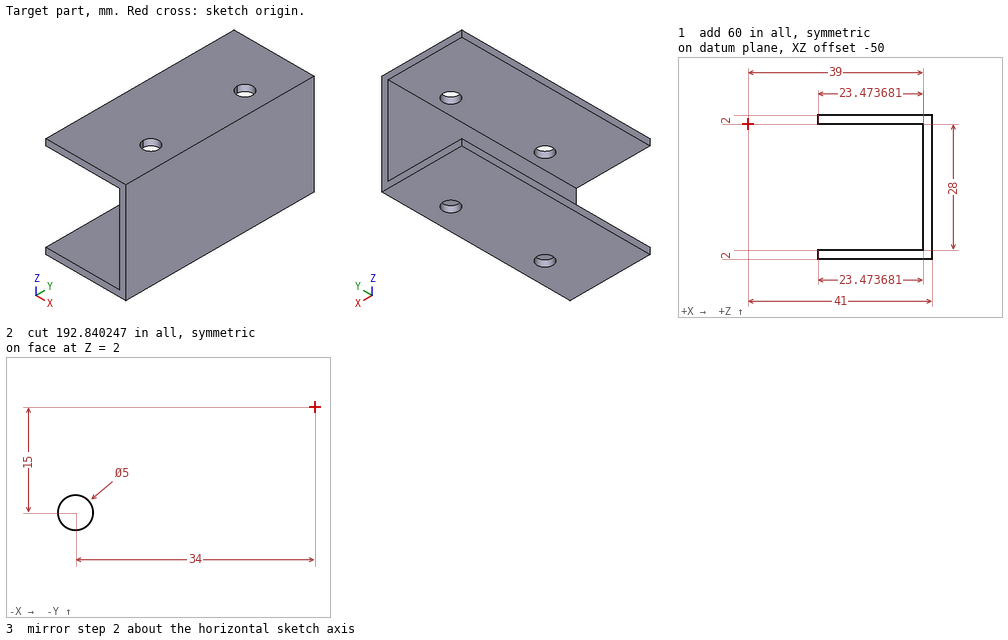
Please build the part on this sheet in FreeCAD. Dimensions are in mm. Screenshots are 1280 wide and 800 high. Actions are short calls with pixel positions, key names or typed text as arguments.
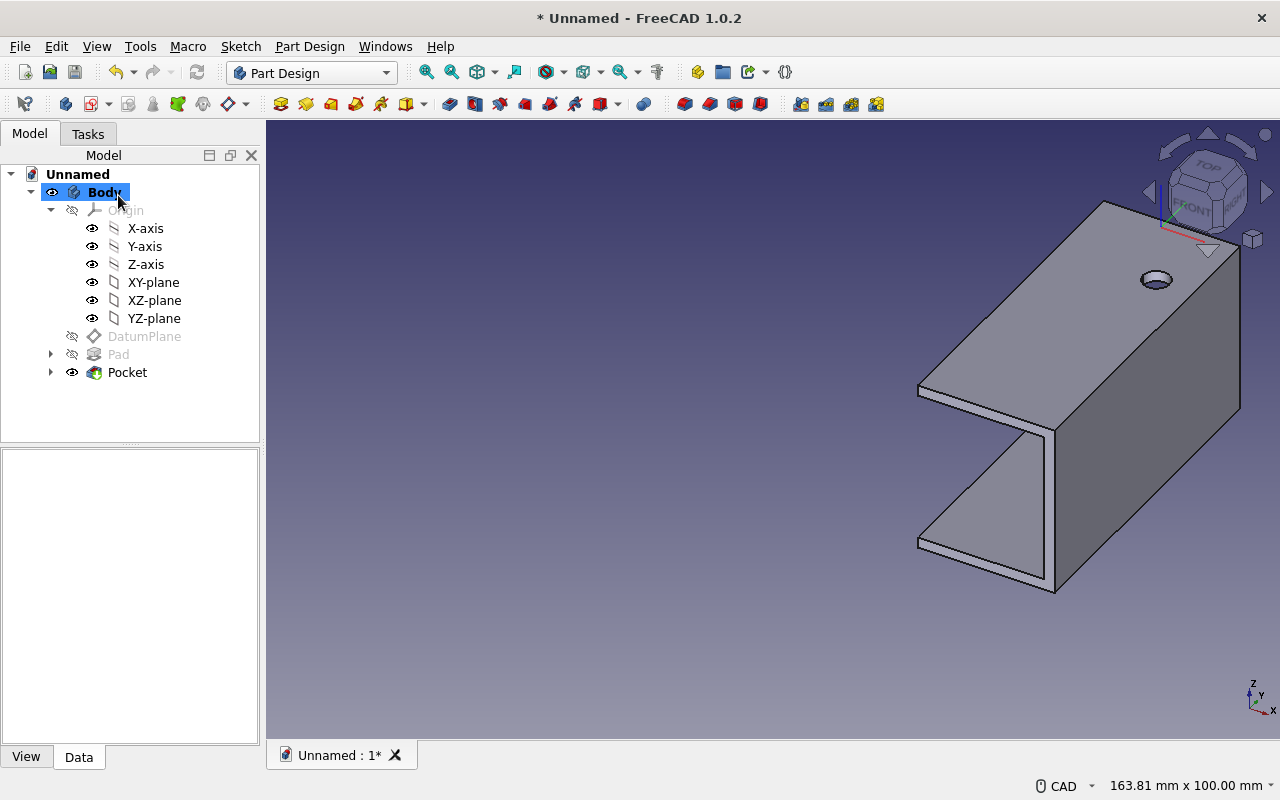
click(117, 372)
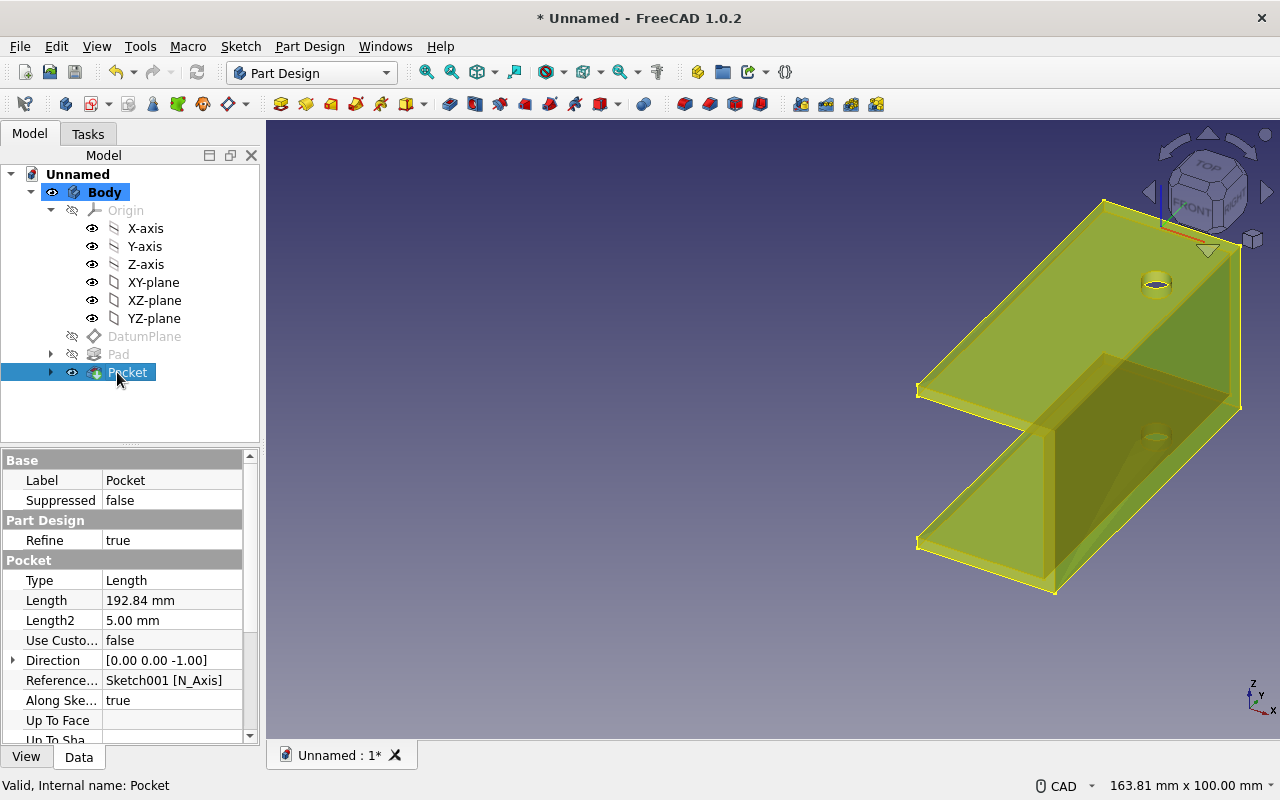
click(801, 104)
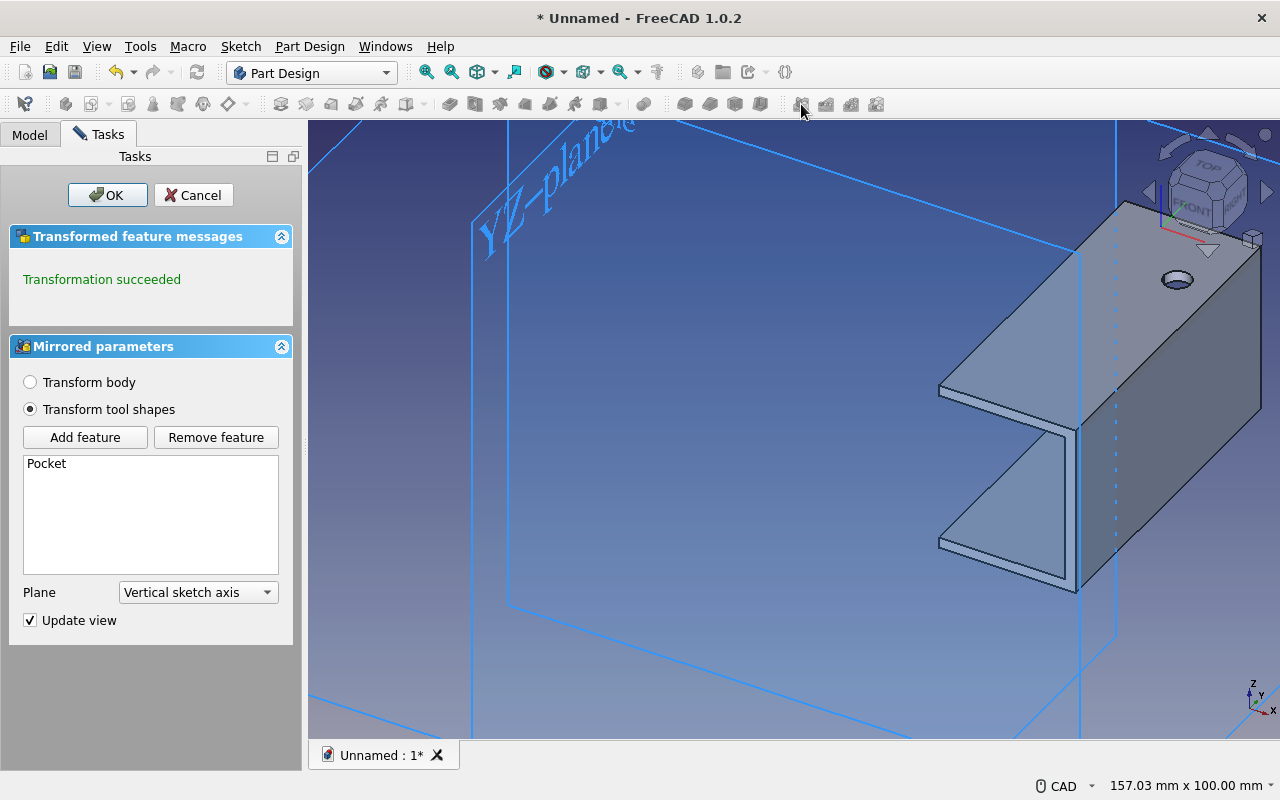
click(199, 592)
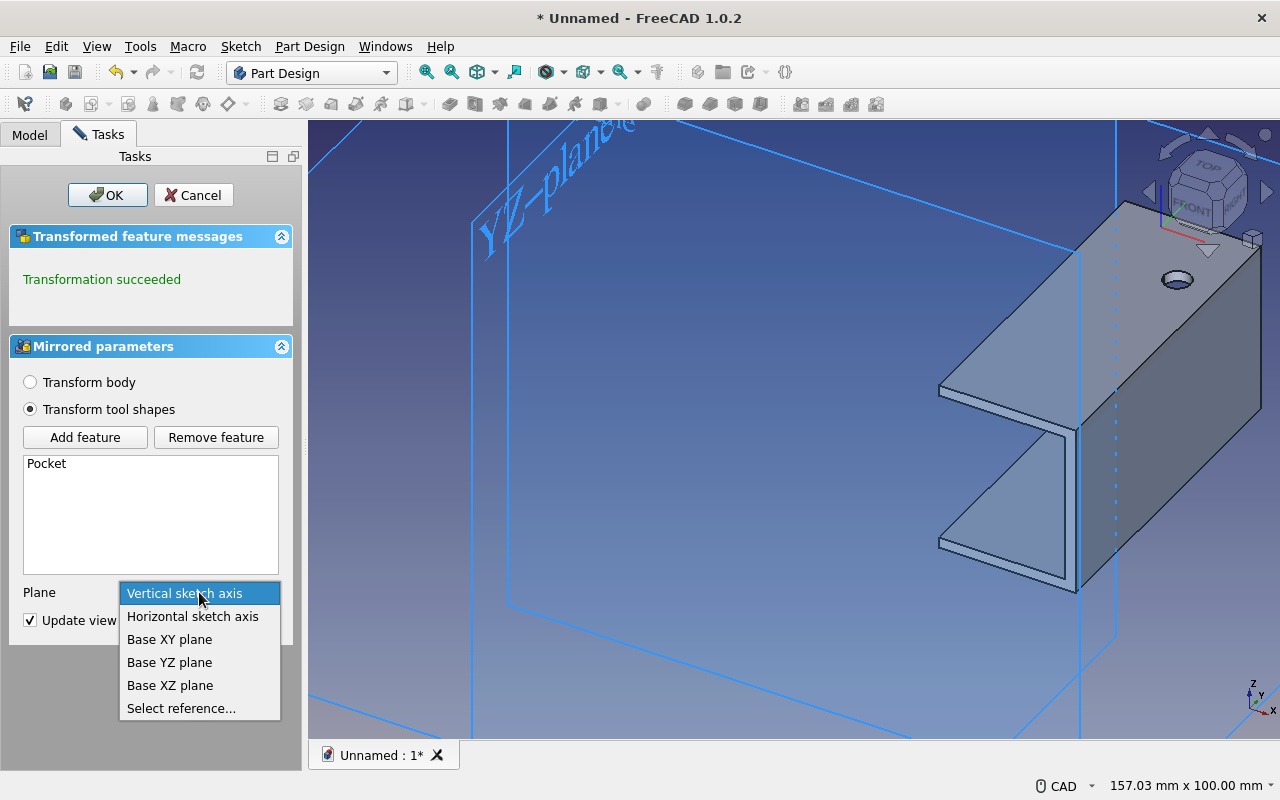
click(198, 616)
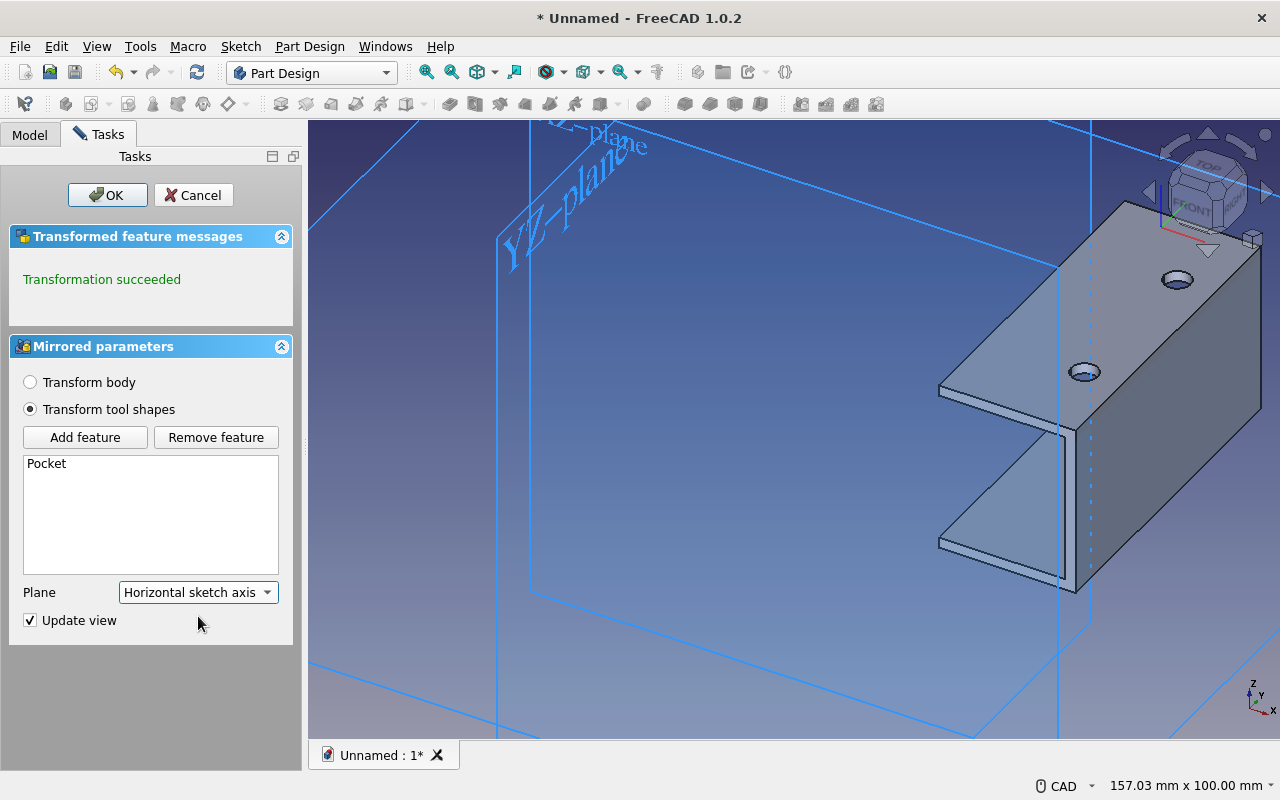
click(108, 195)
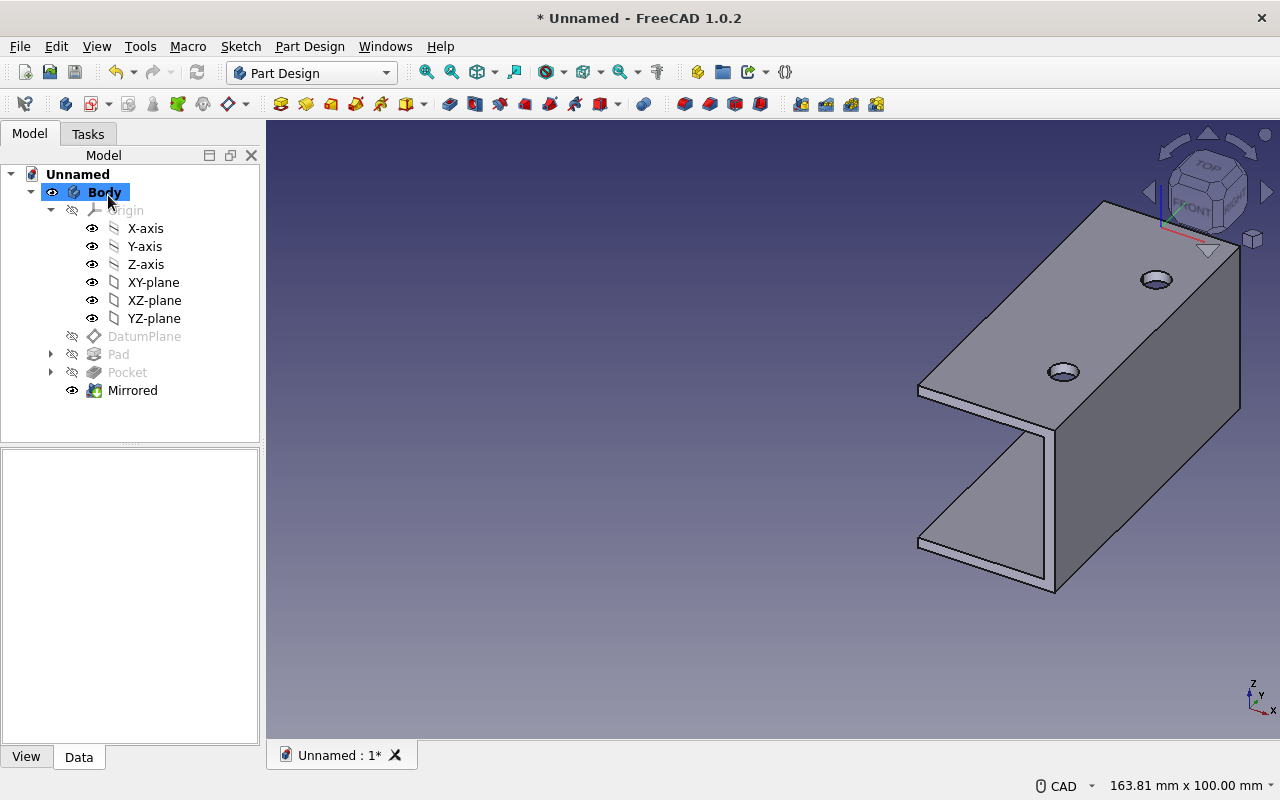
key(0)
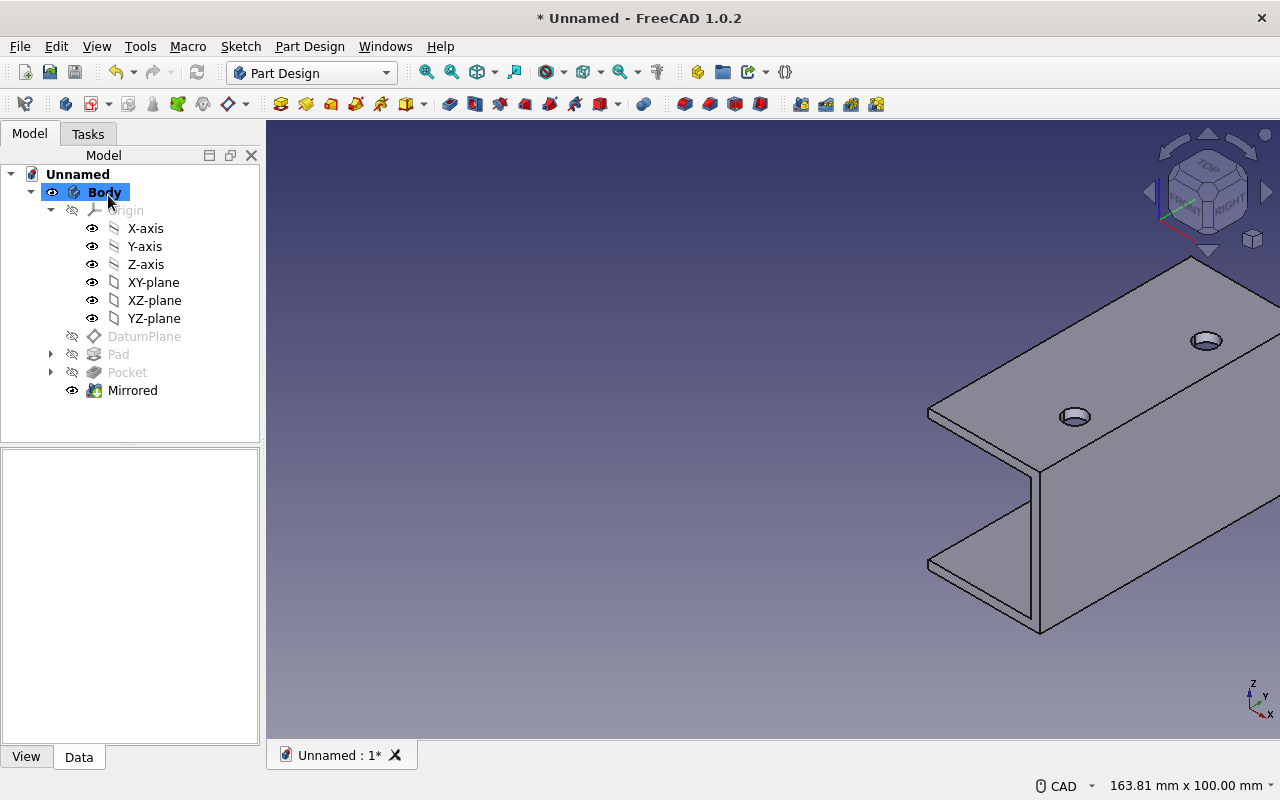
click(427, 72)